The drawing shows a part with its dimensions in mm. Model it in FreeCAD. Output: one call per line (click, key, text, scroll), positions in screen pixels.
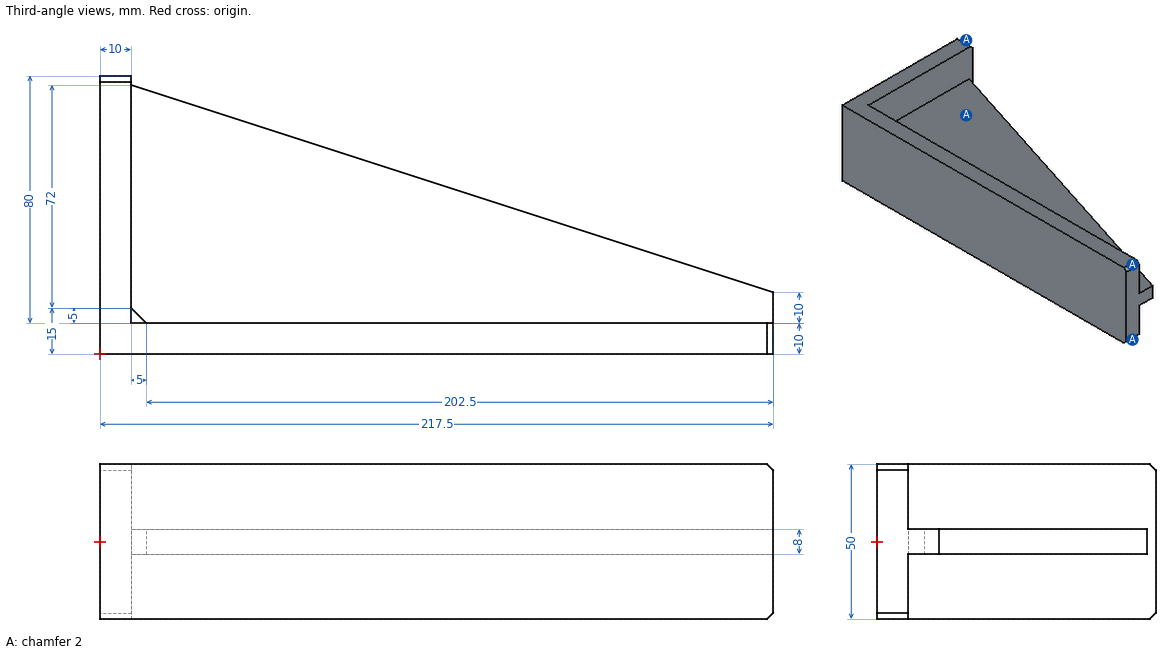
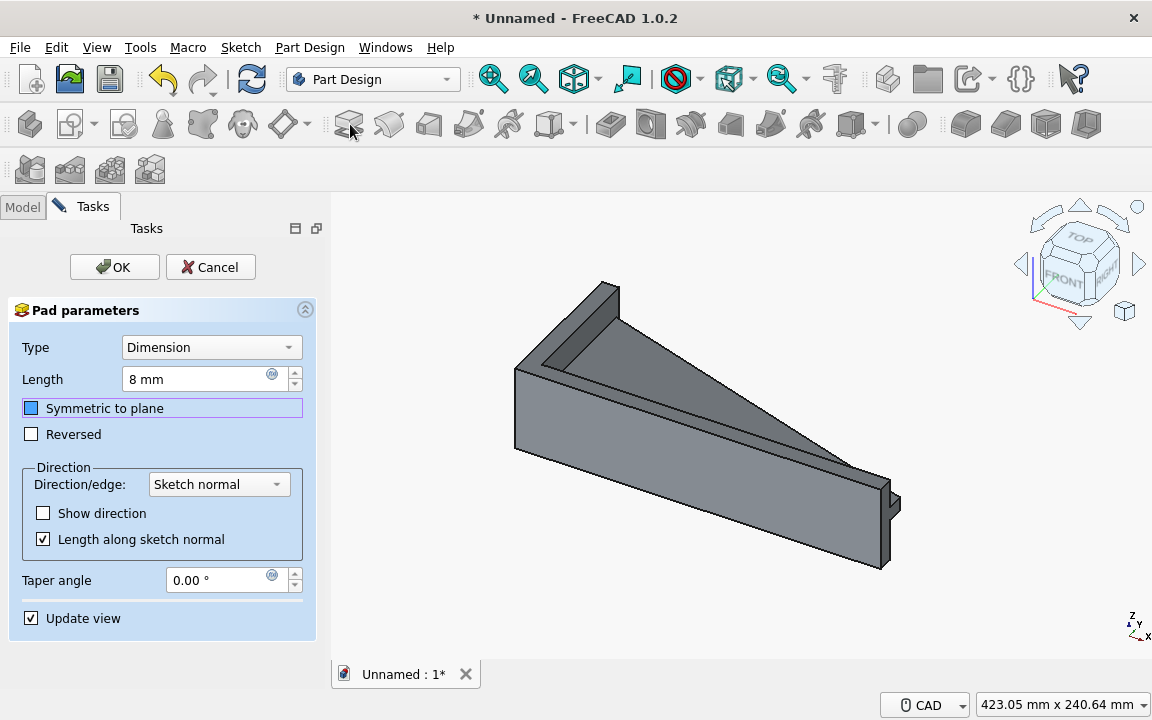
click(30, 408)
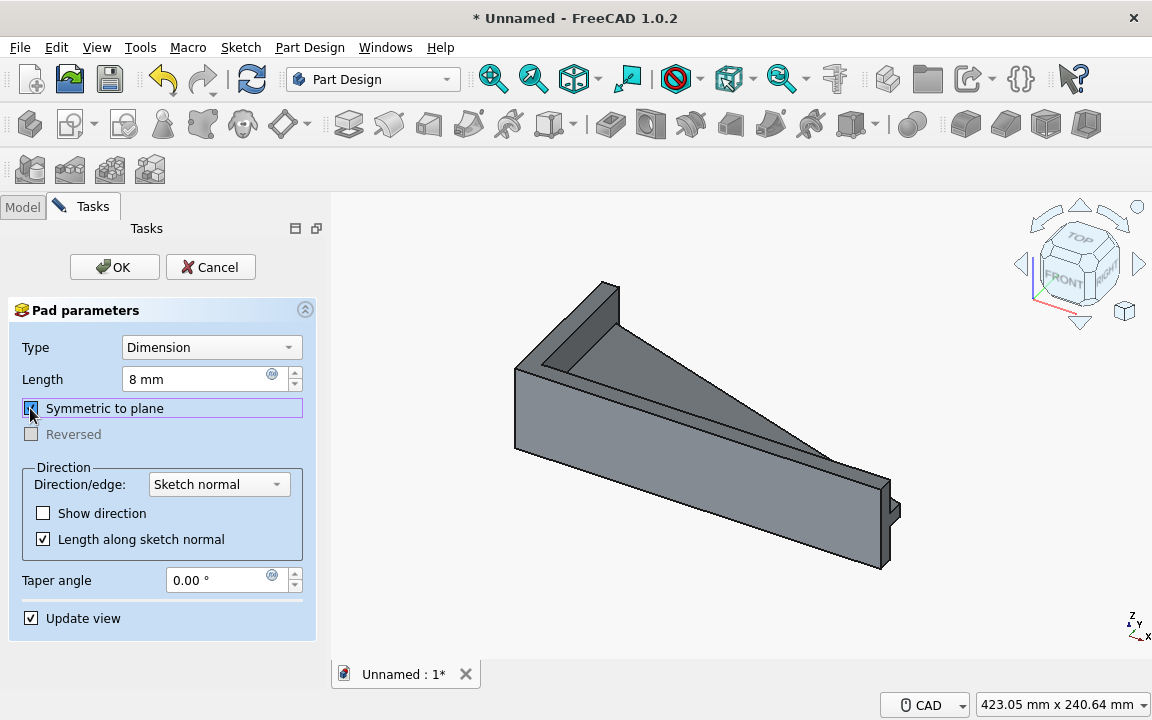
click(115, 267)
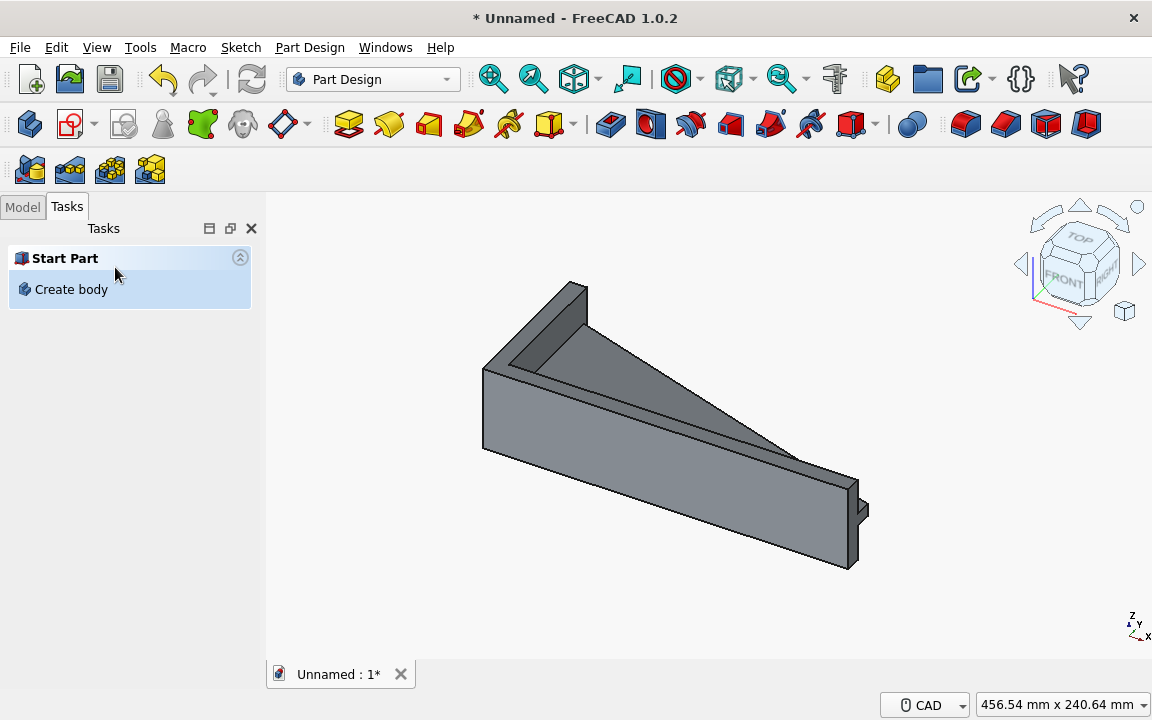
click(853, 484)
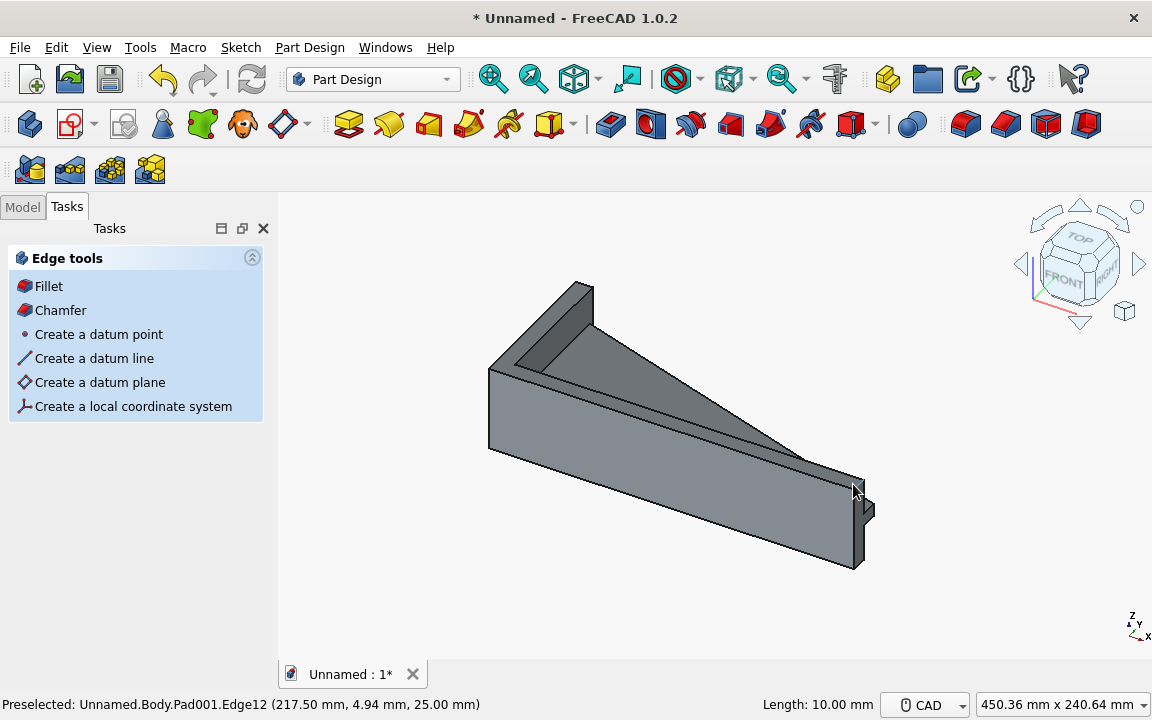
scroll(584, 284, up, 4)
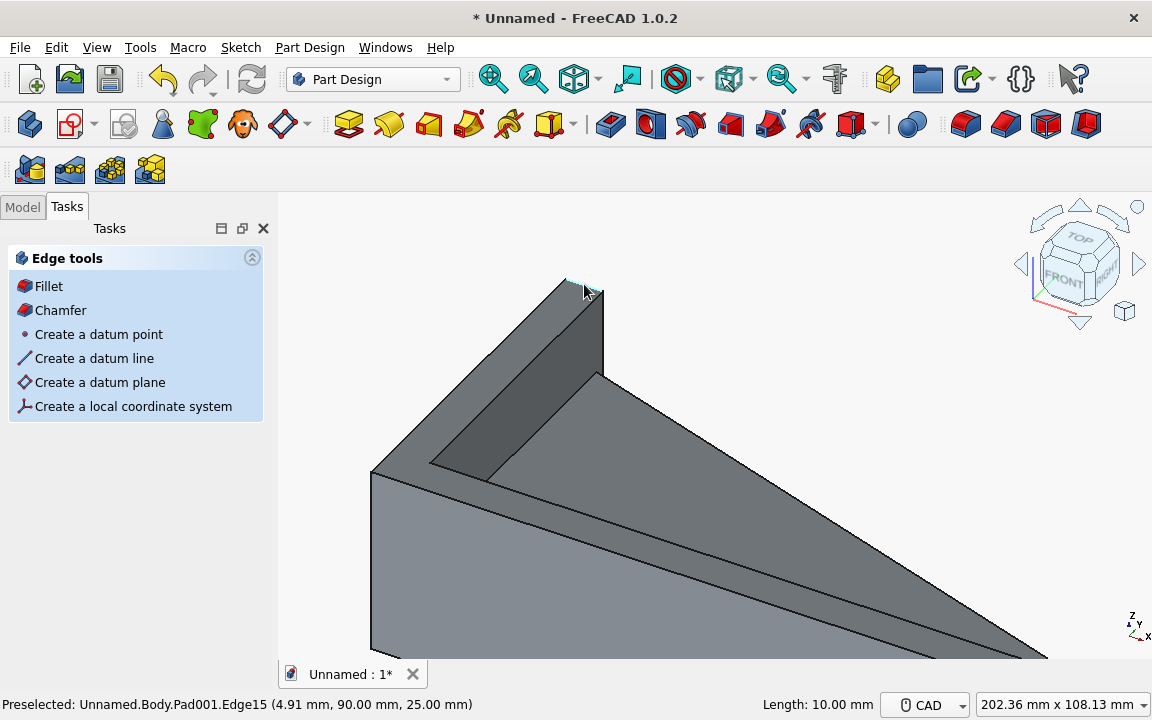
click(494, 80)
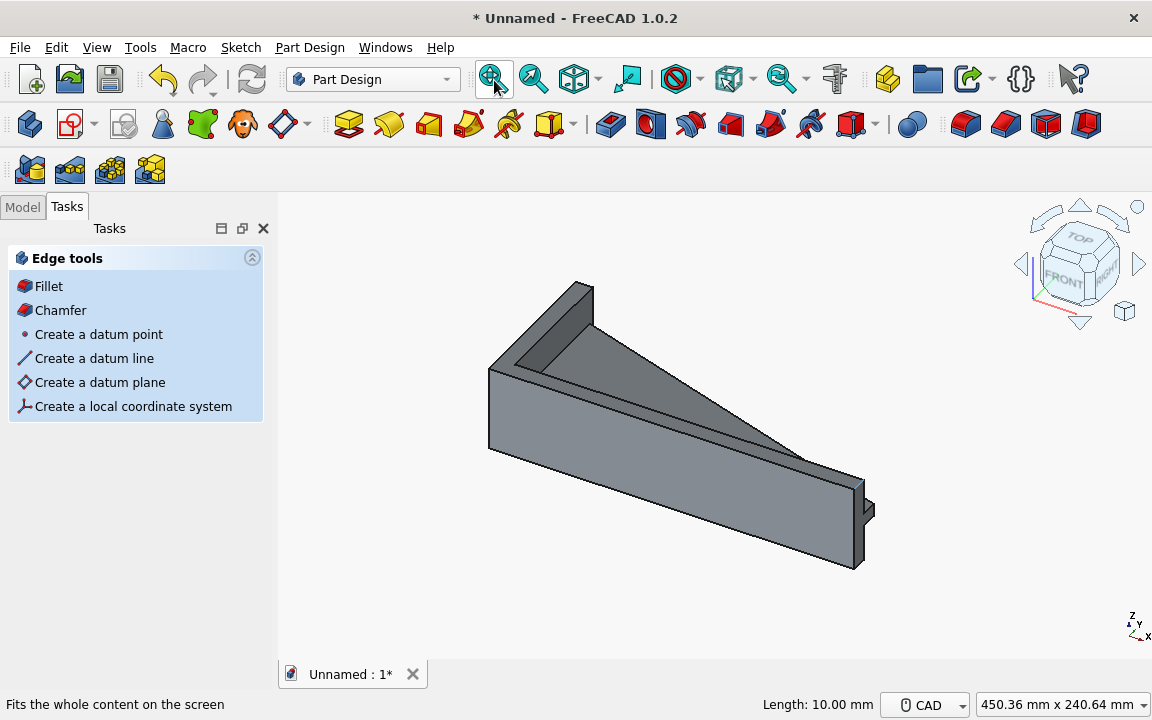
key(0)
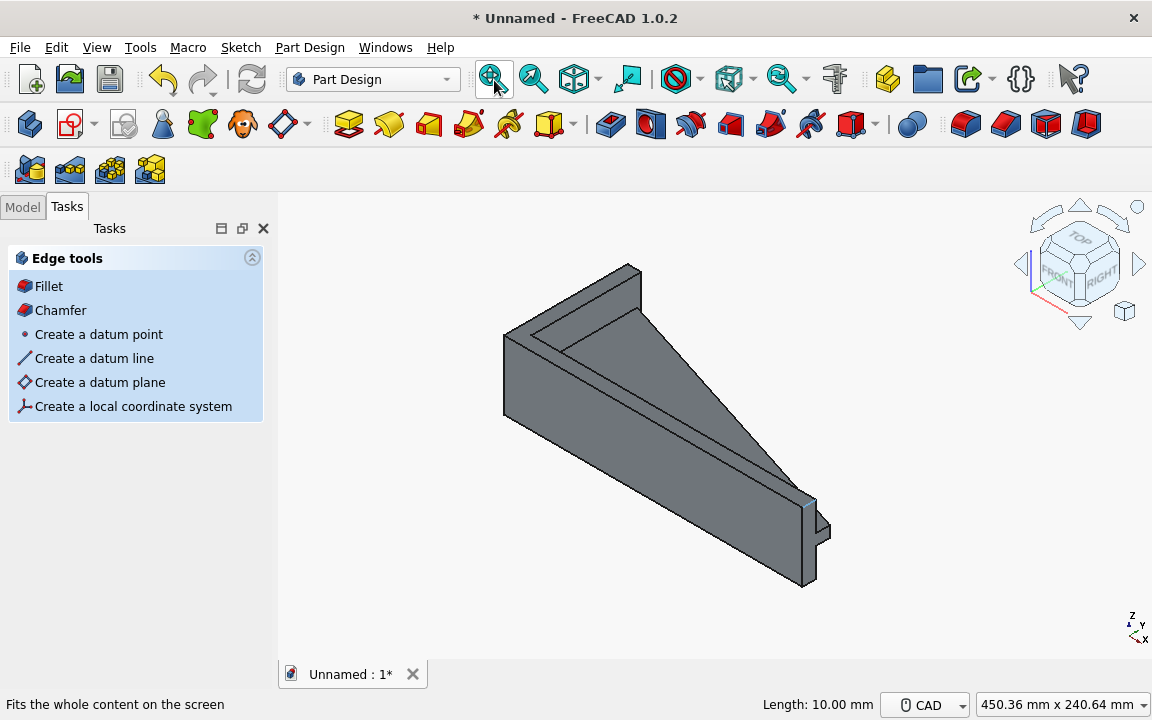
scroll(634, 267, up, 4)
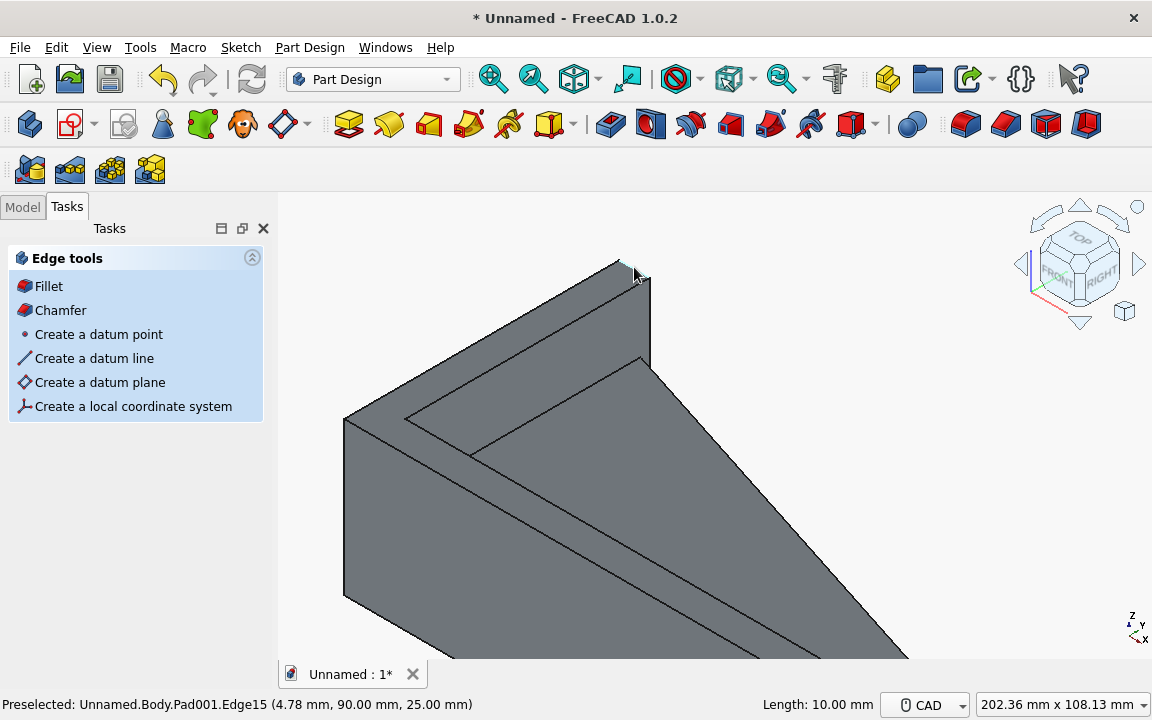
click(494, 80)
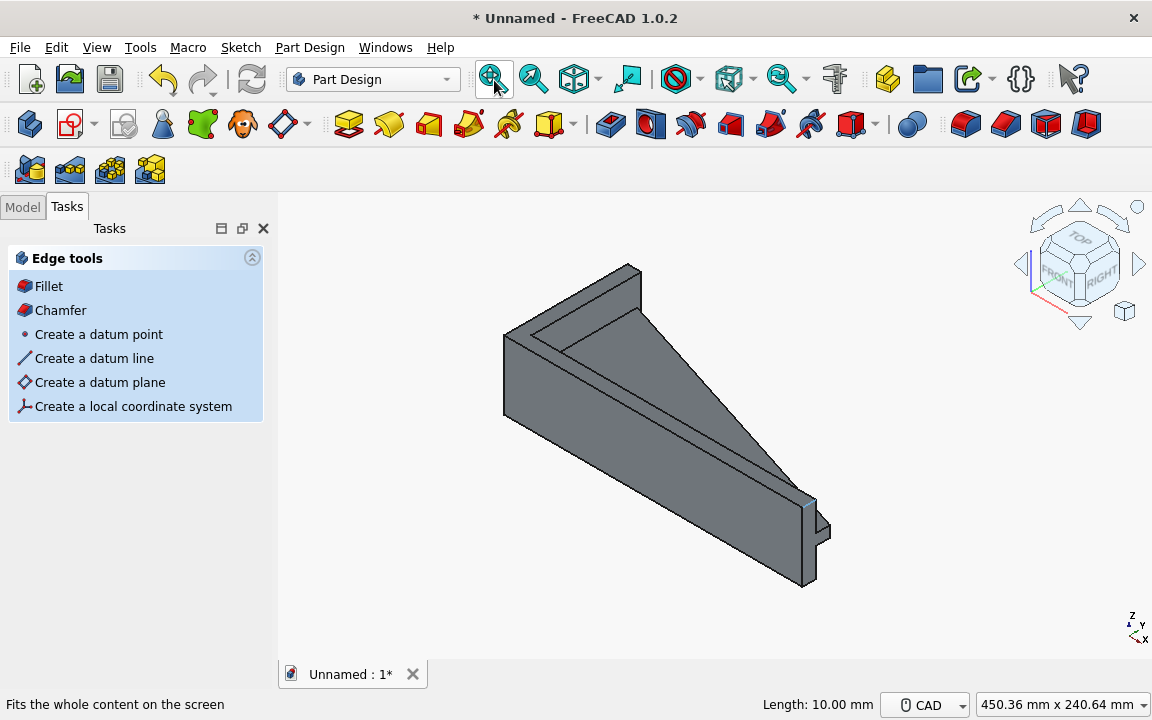
key(2)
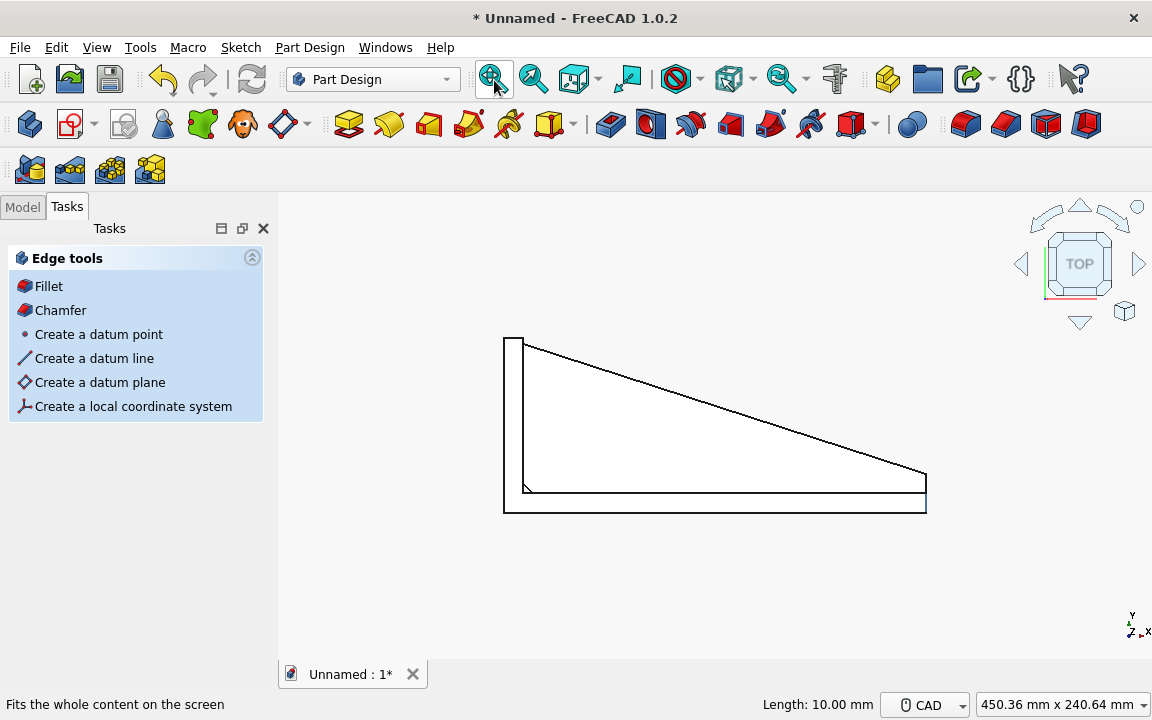
click(514, 337, ctrl)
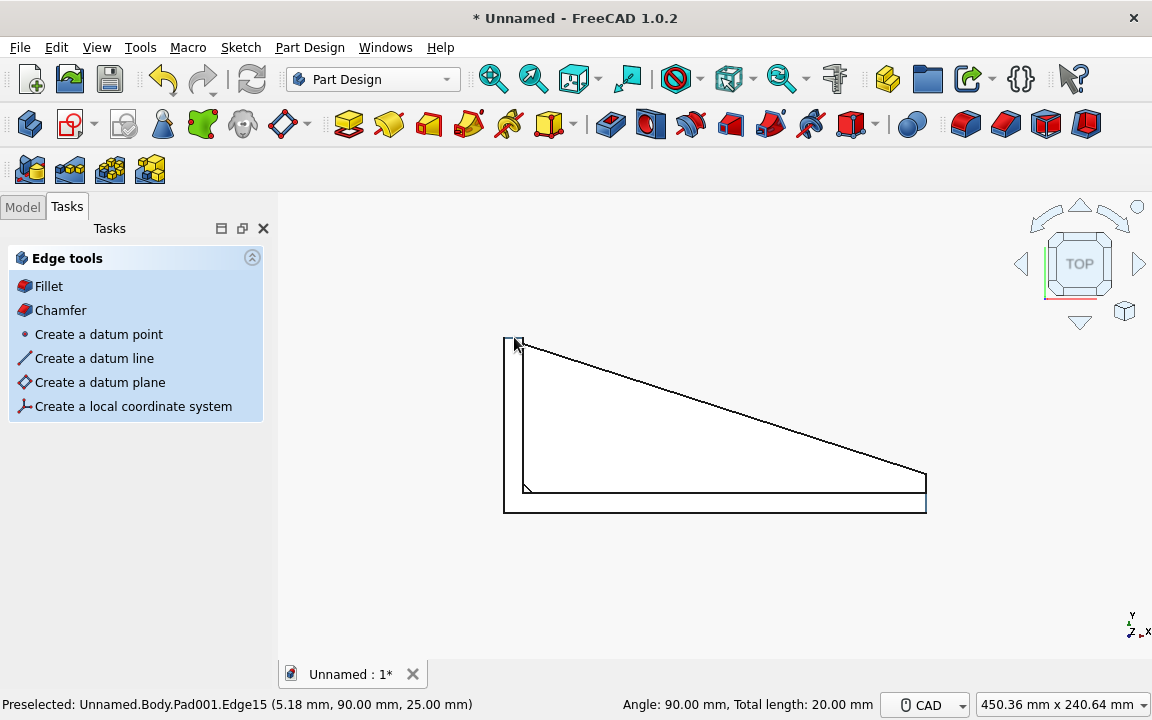
scroll(514, 337, up, 4)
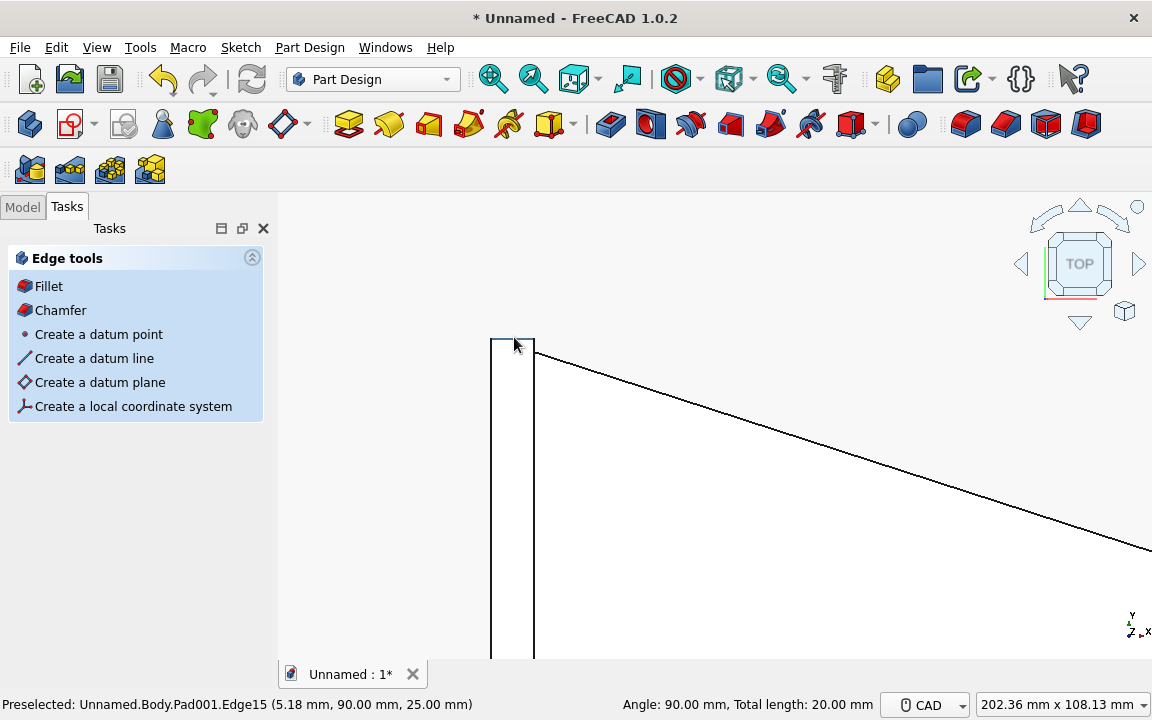
click(494, 80)